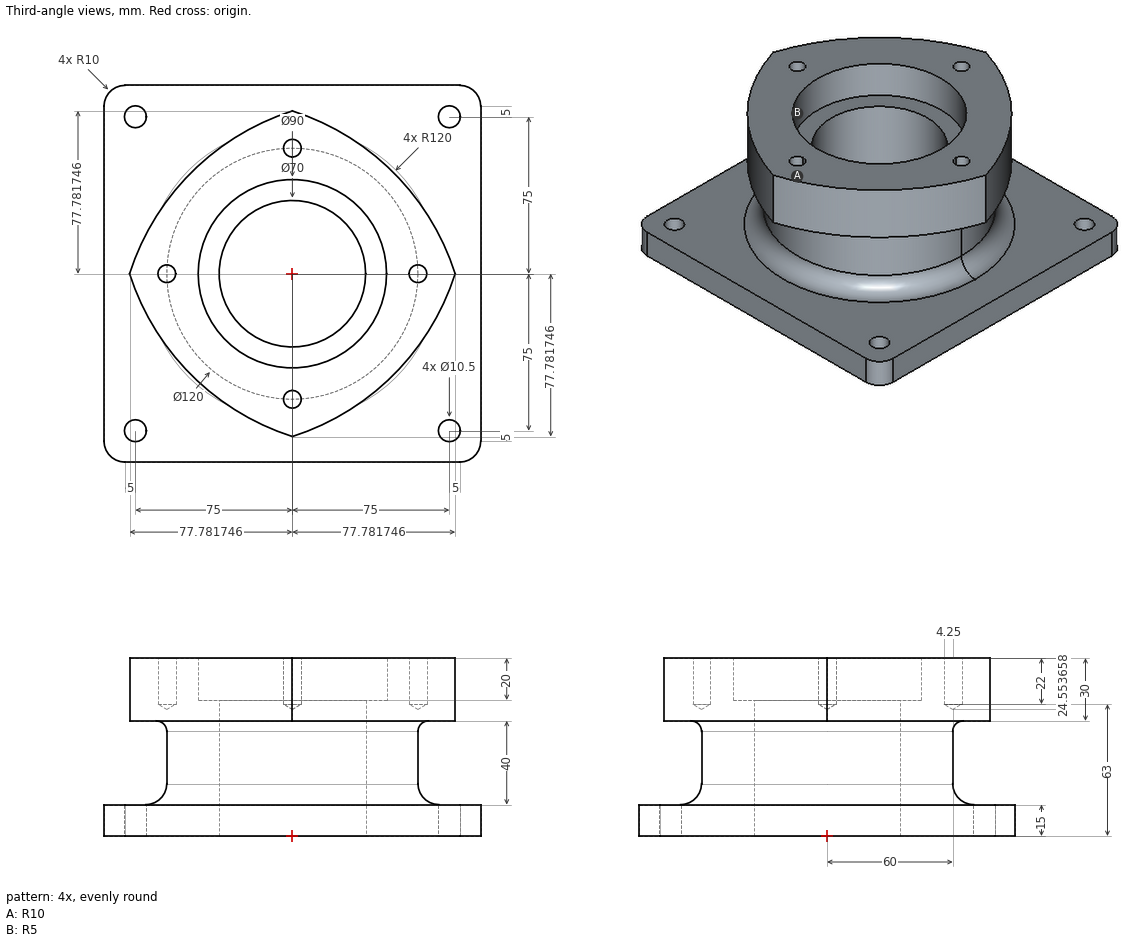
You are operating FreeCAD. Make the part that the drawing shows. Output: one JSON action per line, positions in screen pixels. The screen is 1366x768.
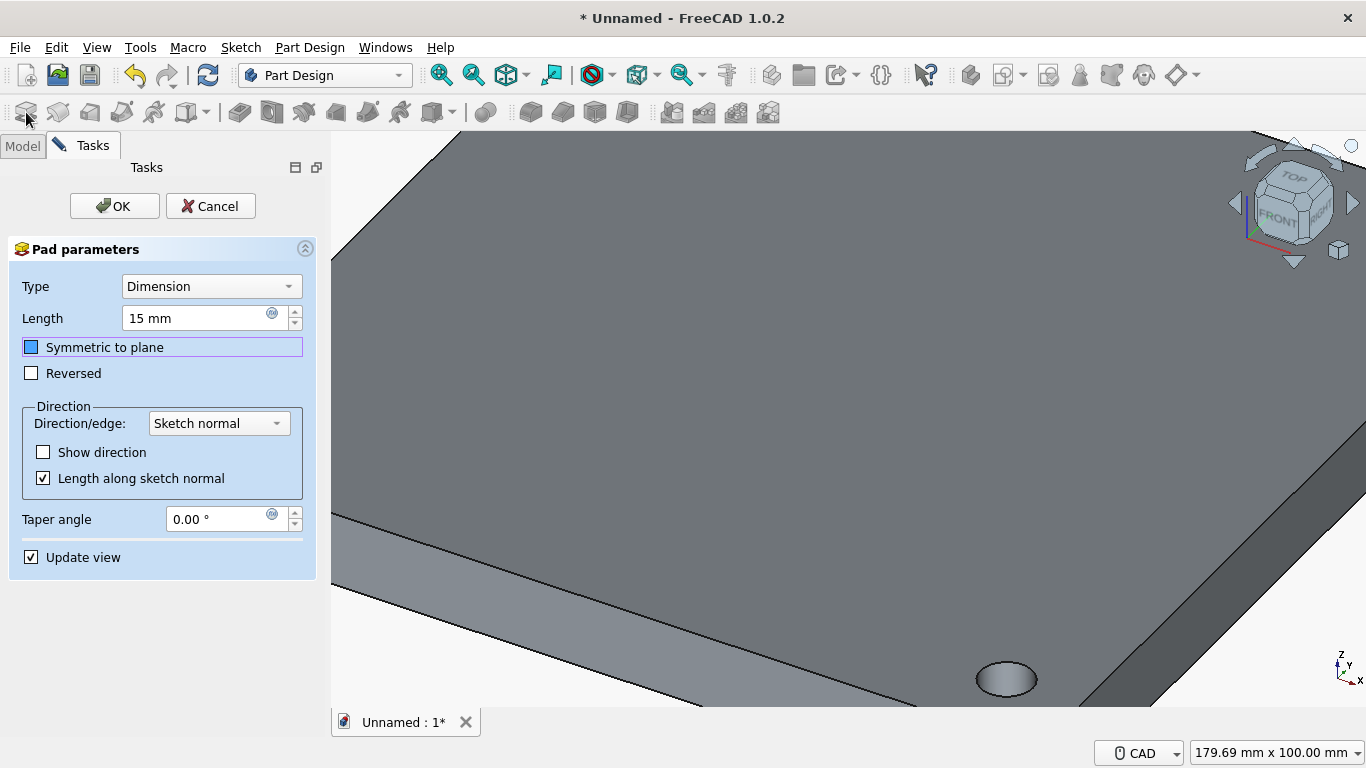
{"action": "left_click", "coordinate": [115, 206]}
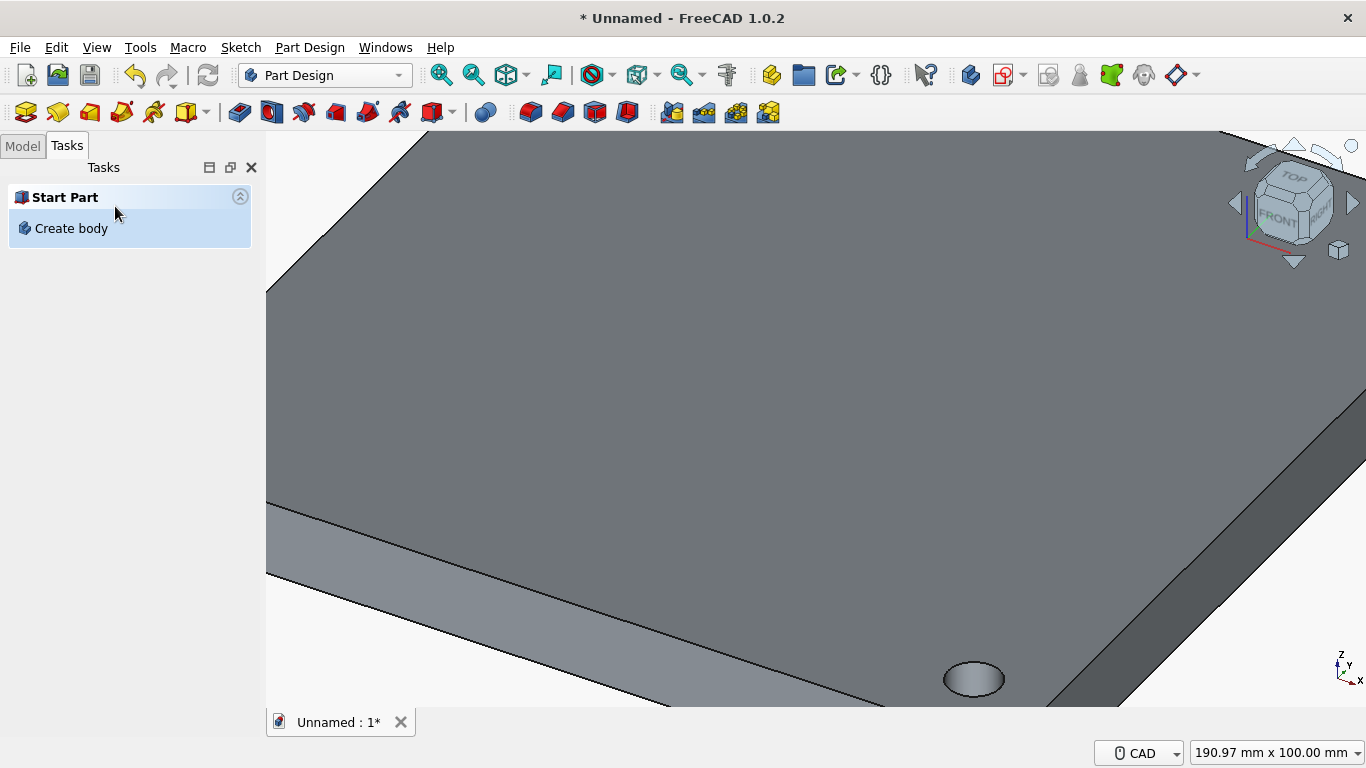
{"action": "left_click", "coordinate": [442, 76]}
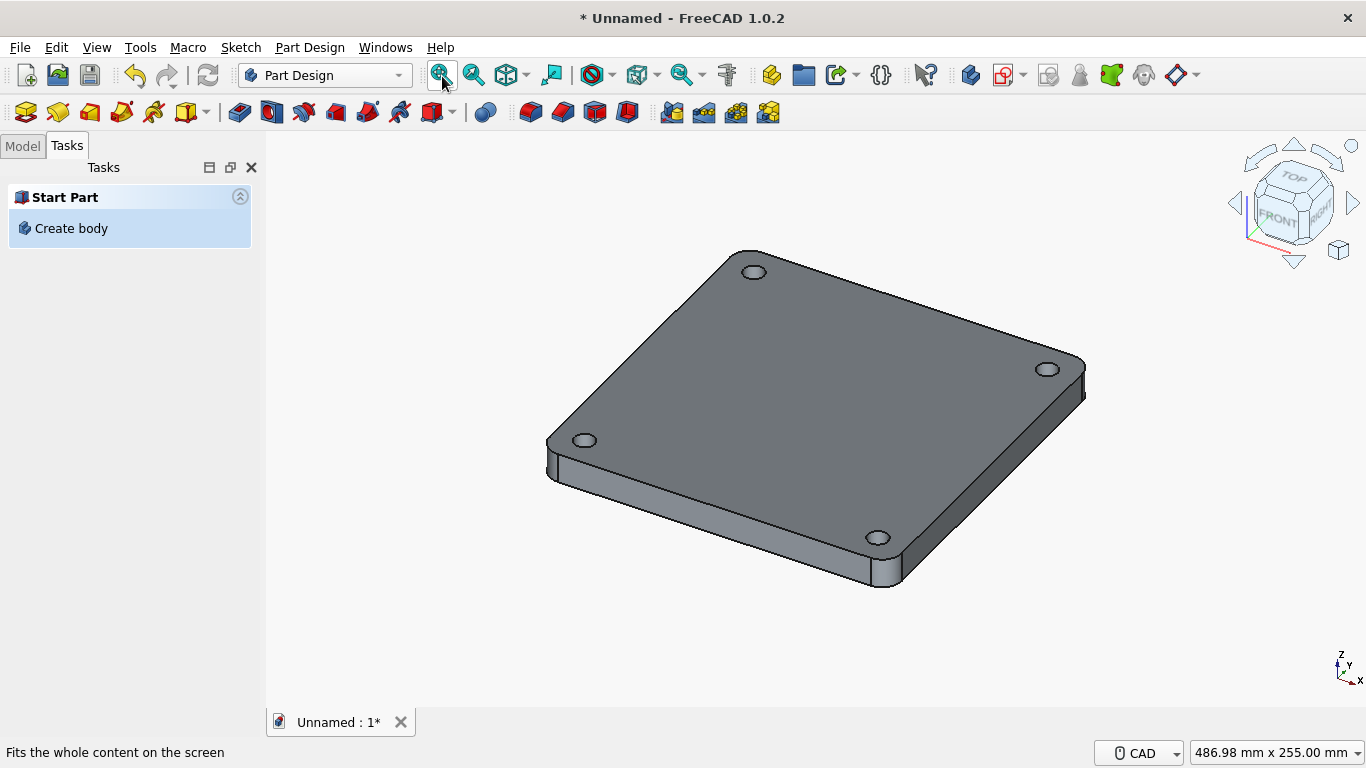
{"action": "left_click", "coordinate": [816, 404]}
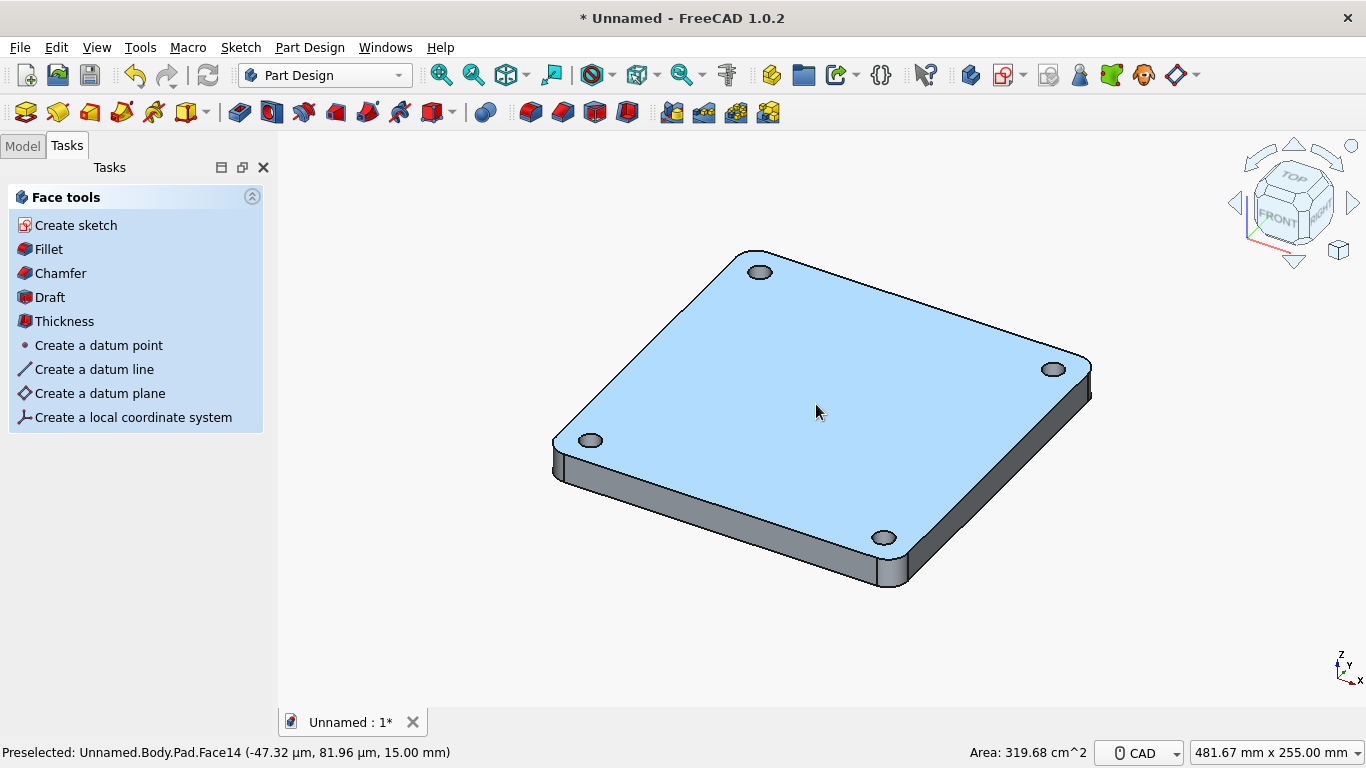
{"action": "left_click", "coordinate": [1004, 76]}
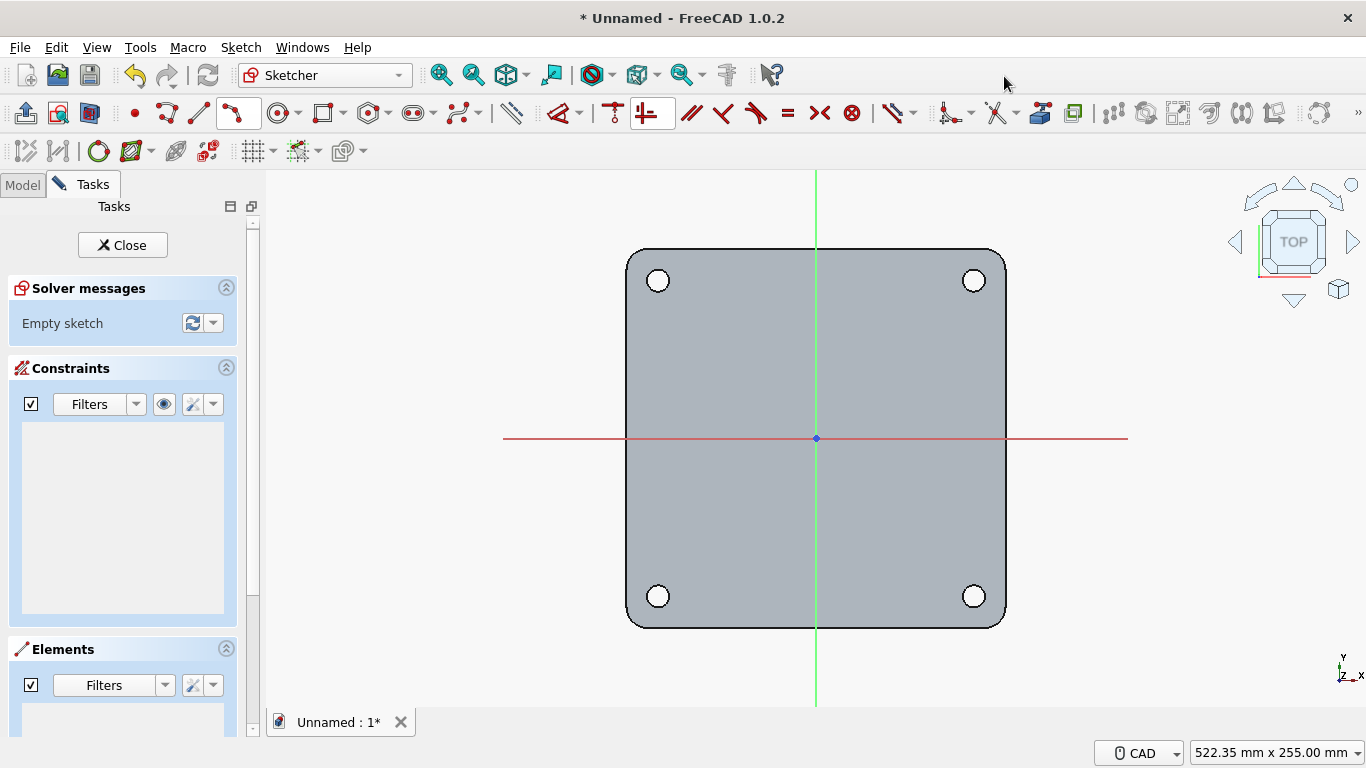
{"action": "left_click", "coordinate": [278, 114]}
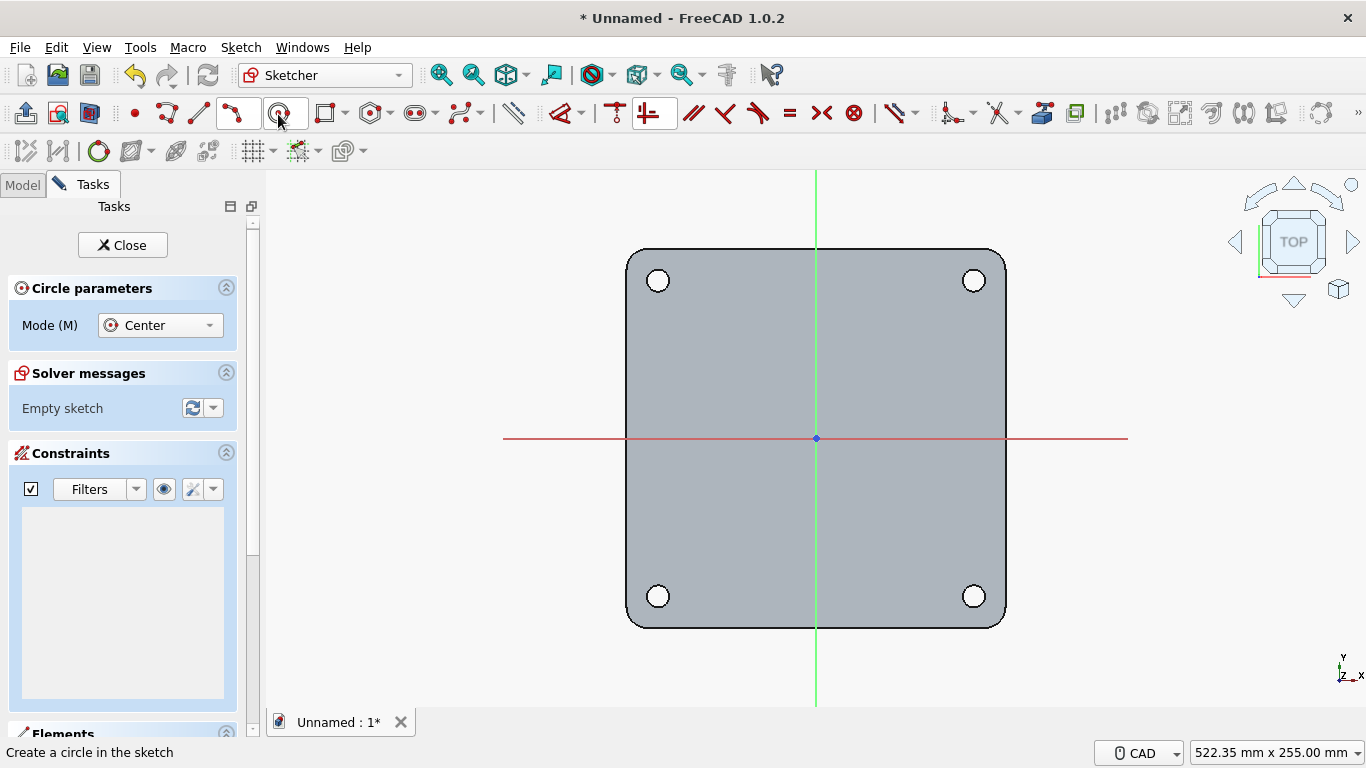
{"action": "left_click", "coordinate": [816, 438]}
{"action": "mouse_move", "coordinate": [905, 349]}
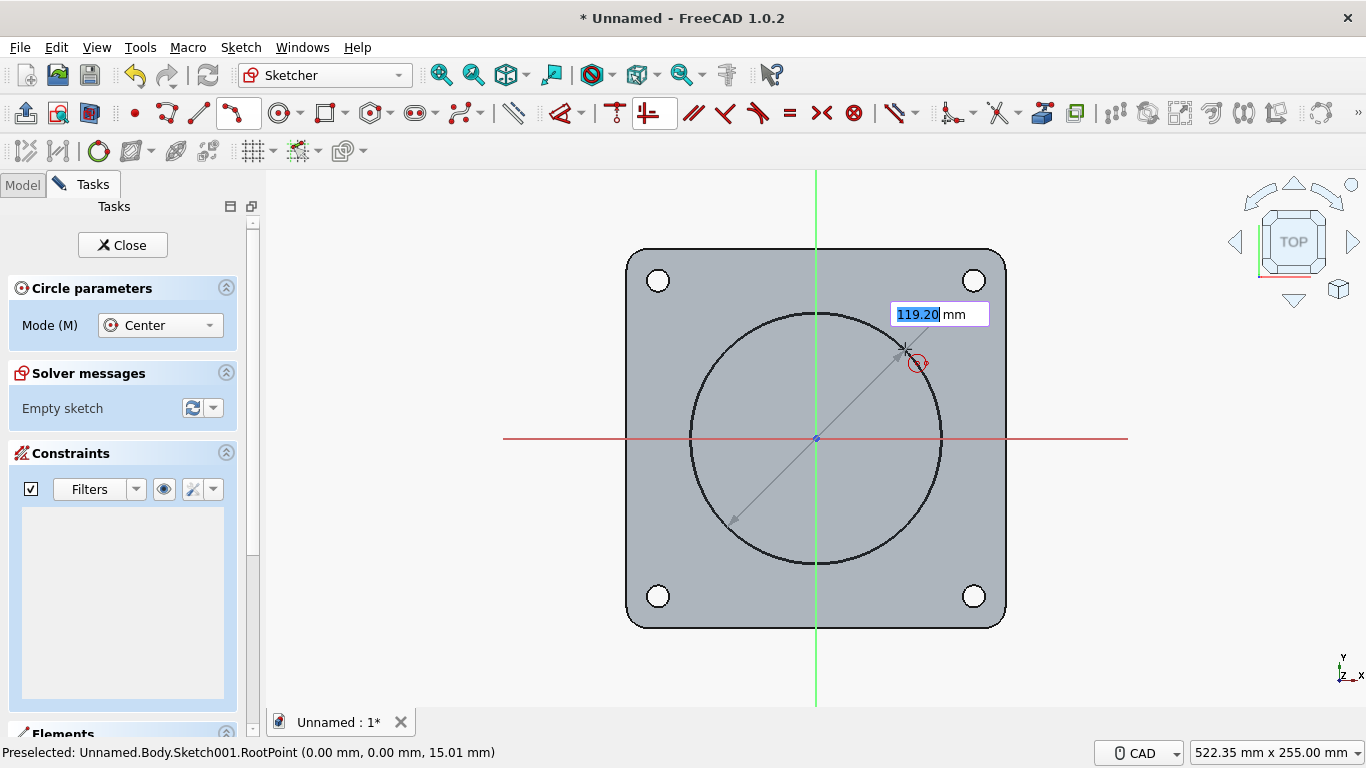
{"action": "type", "text": "120"}
{"action": "key", "text": "Return"}
{"action": "key", "text": "Escape"}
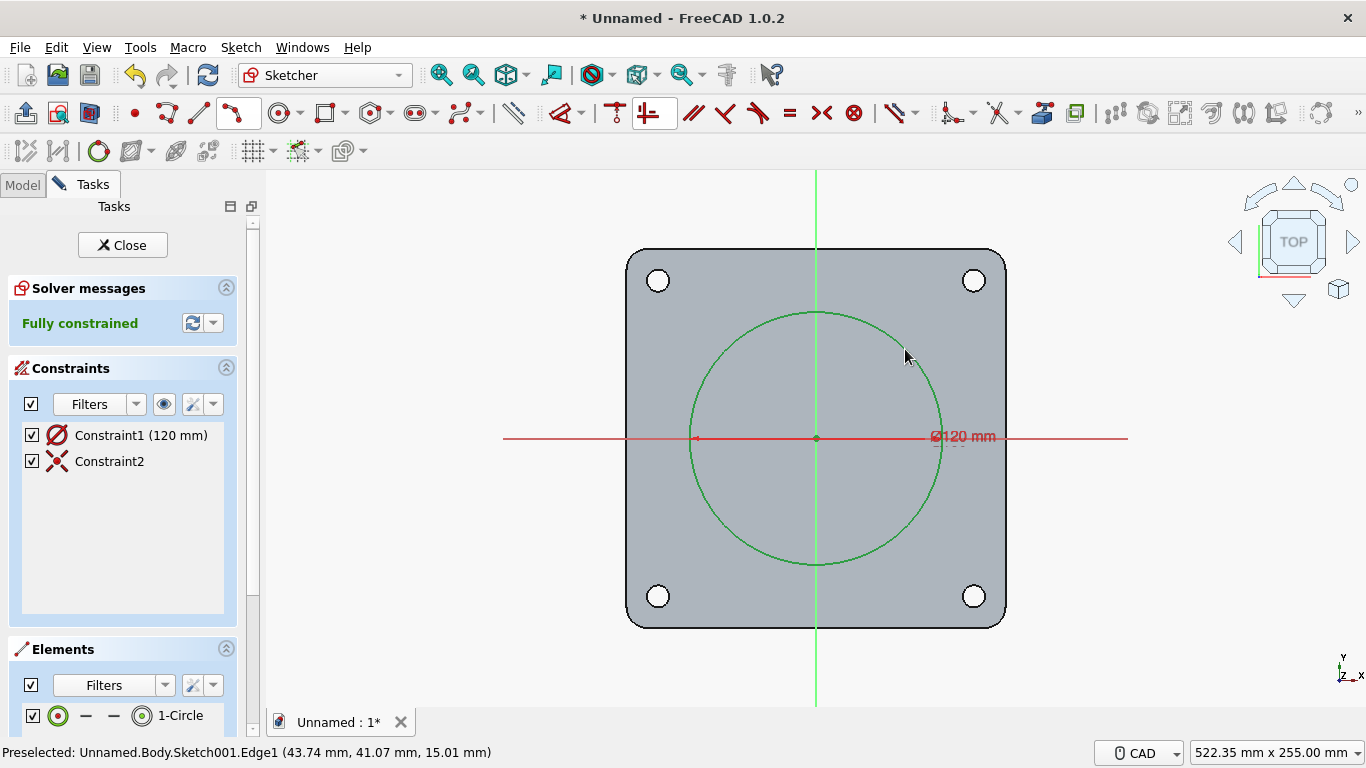
{"action": "left_click", "coordinate": [123, 245]}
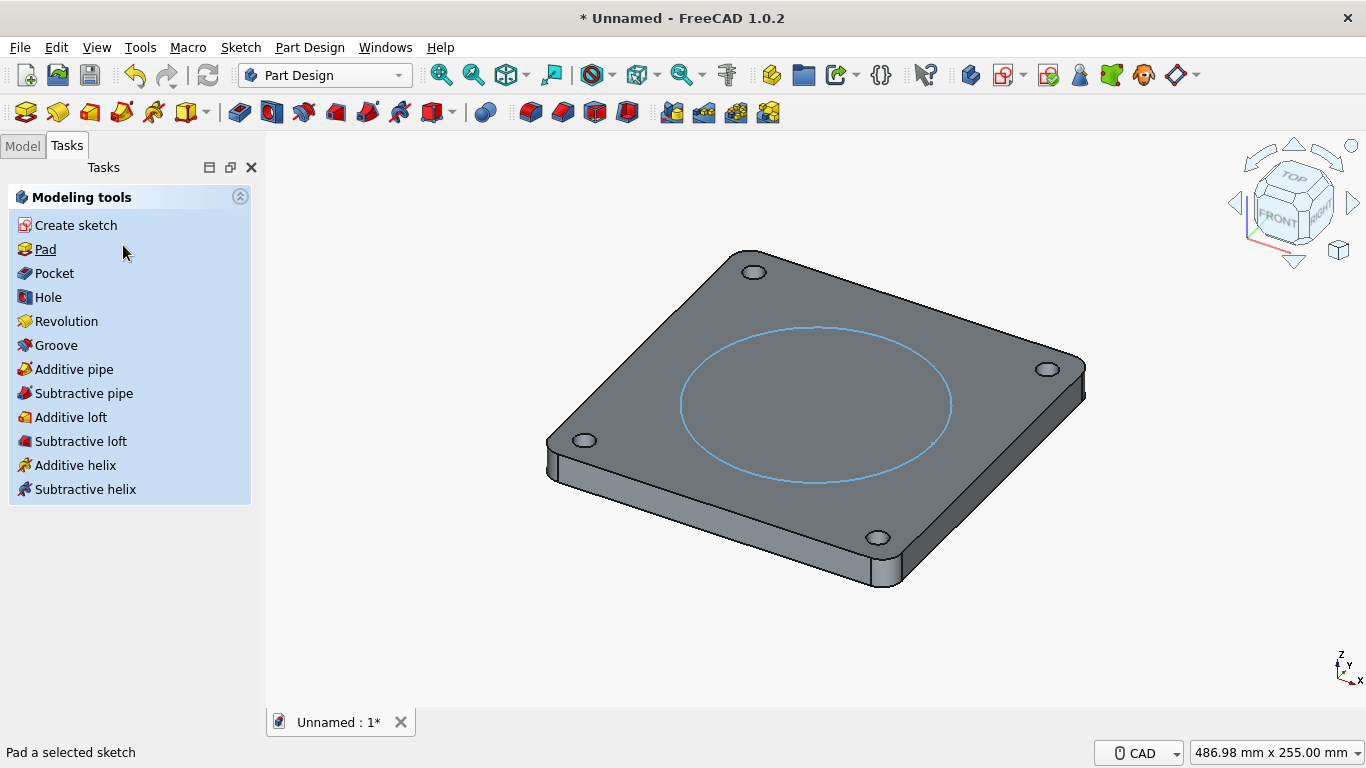
{"action": "left_click", "coordinate": [26, 112]}